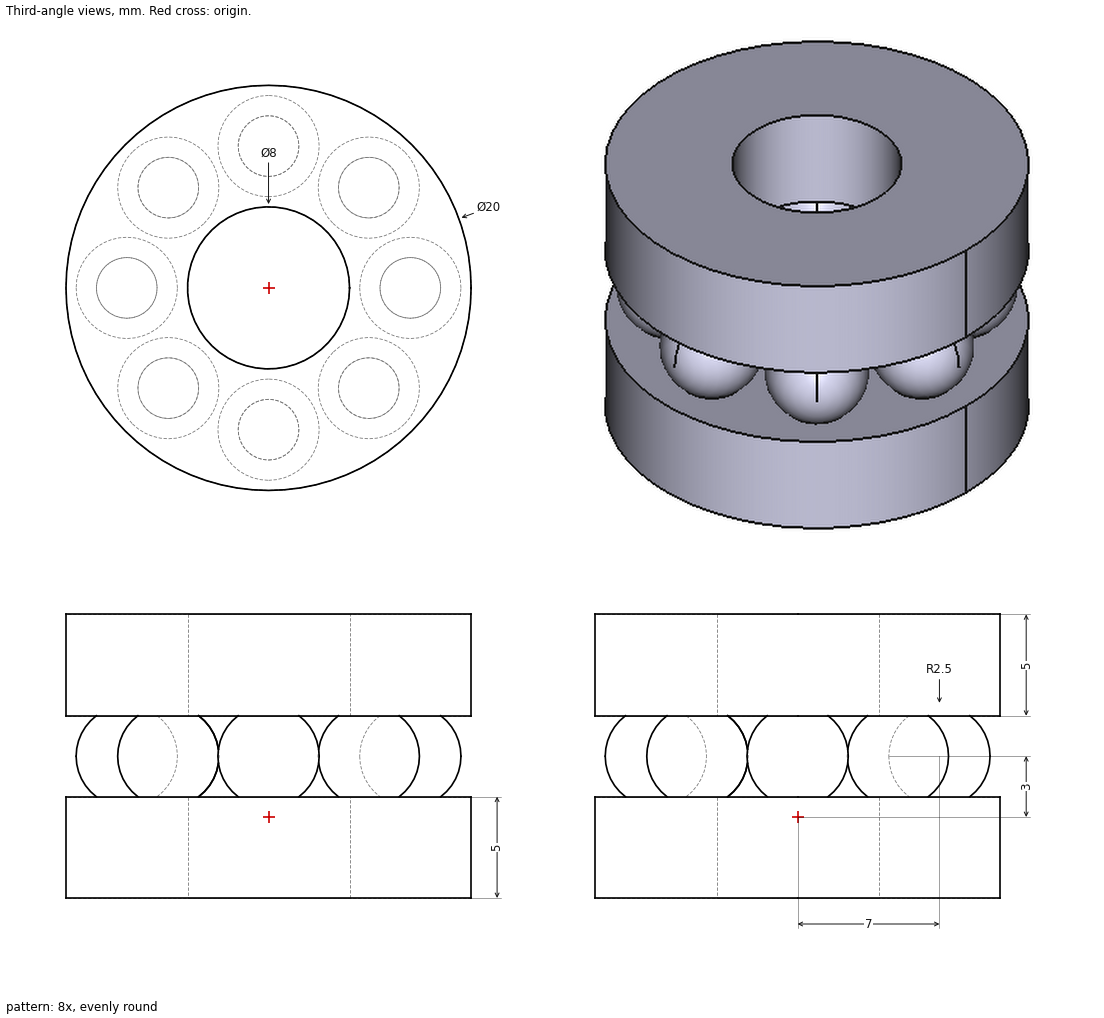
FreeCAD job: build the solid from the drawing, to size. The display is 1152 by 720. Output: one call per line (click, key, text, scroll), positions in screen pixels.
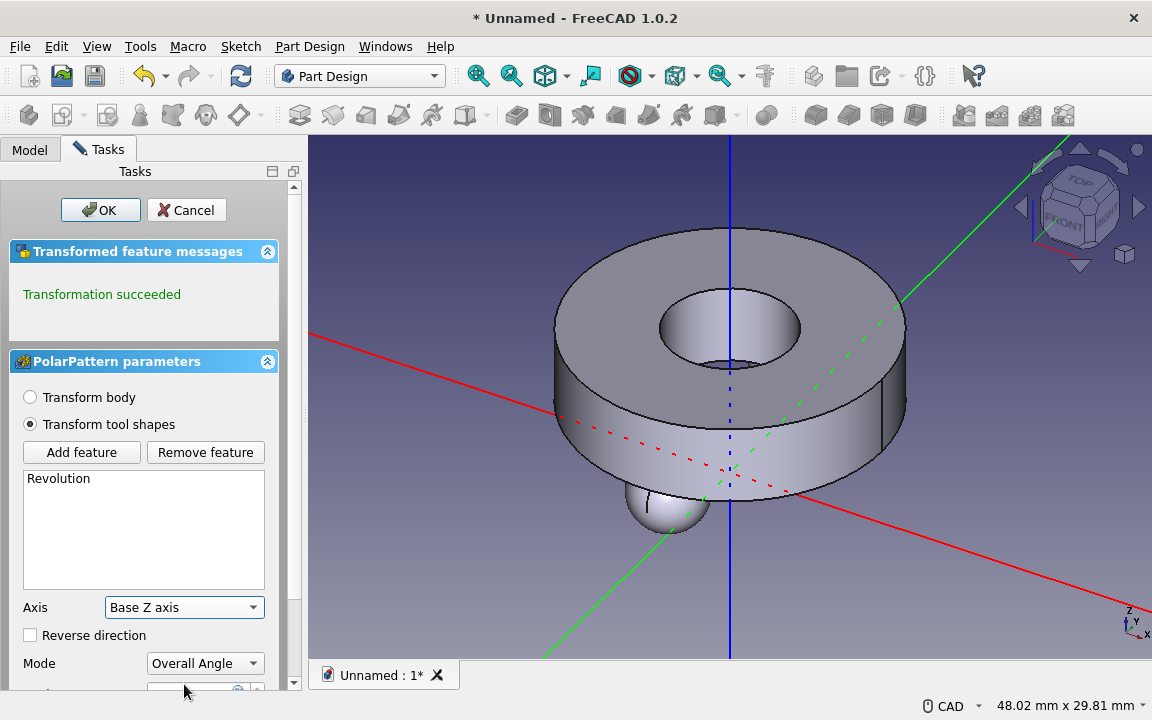
scroll(294, 436, down, 2)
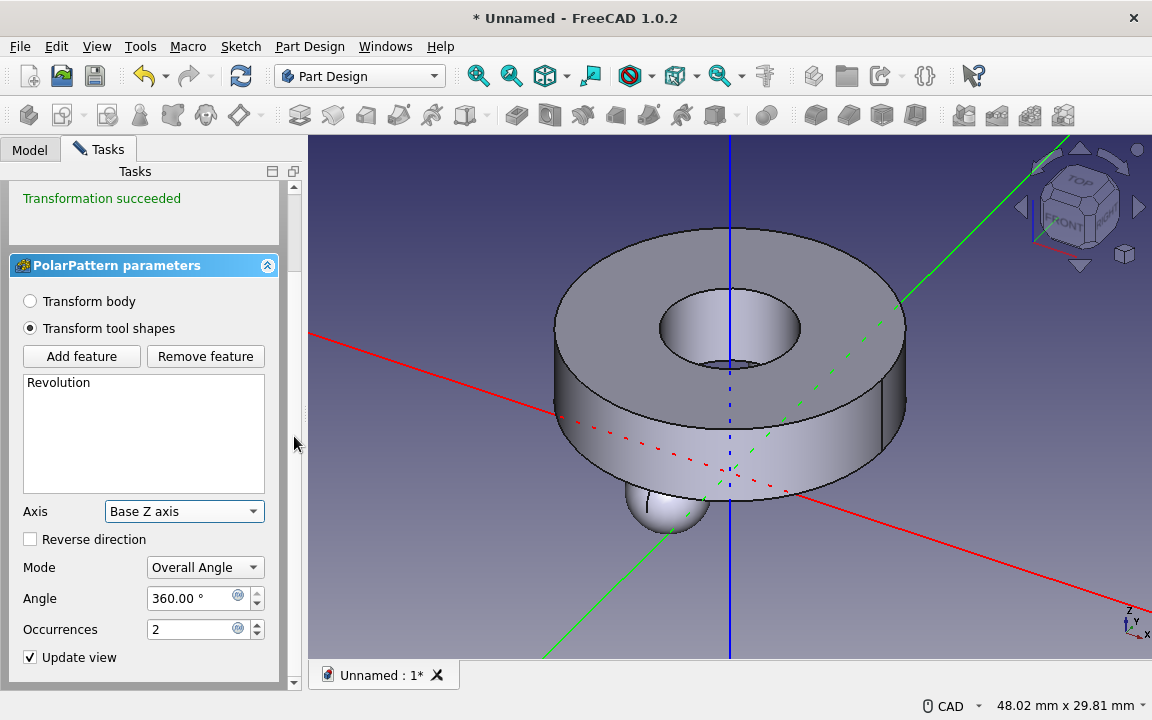
triple_click(199, 630)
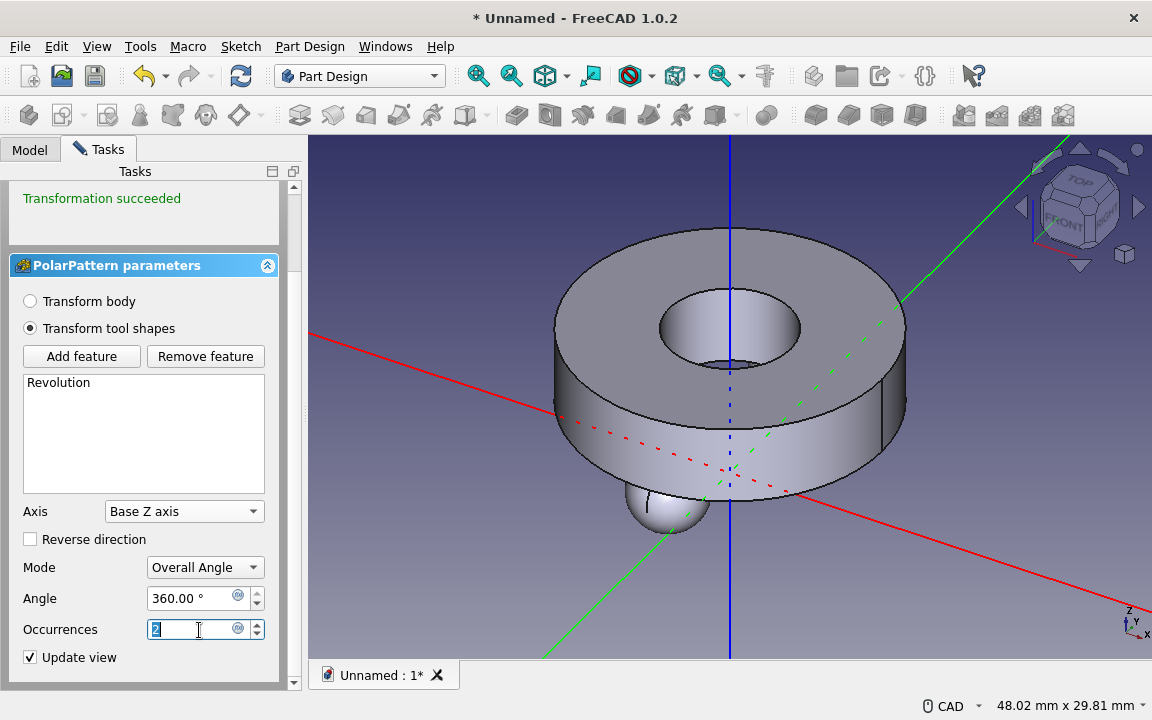
text(8)
key(Tab)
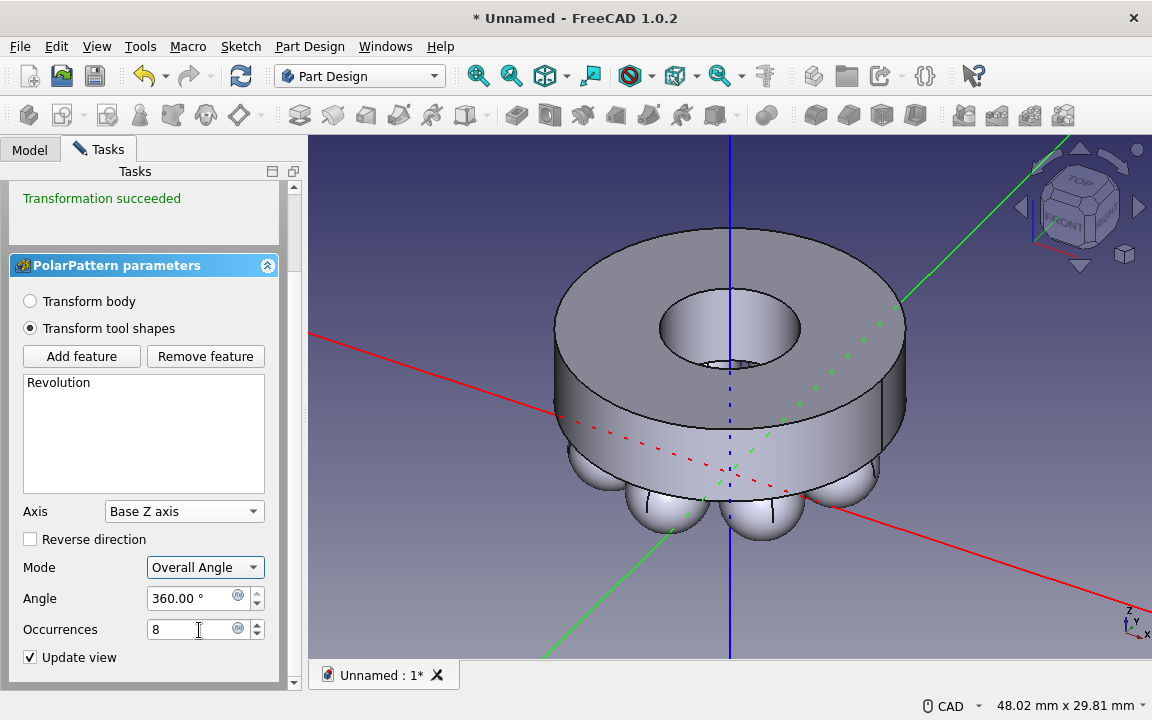
scroll(294, 436, up, 3)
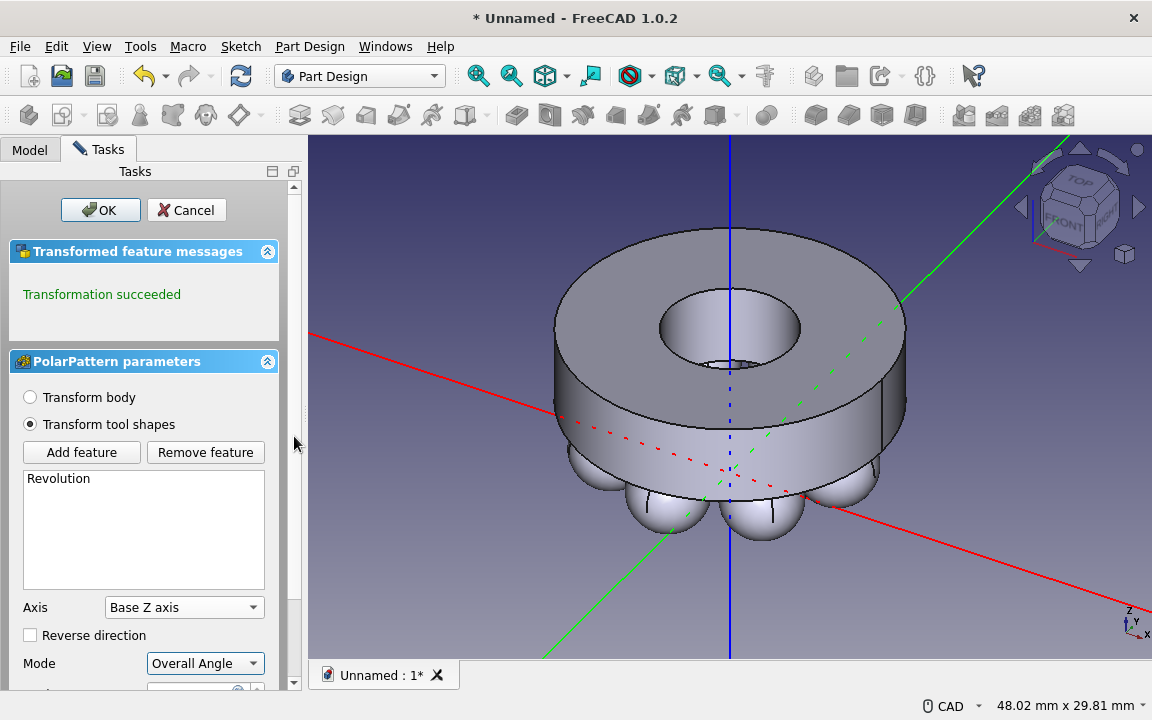
click(101, 210)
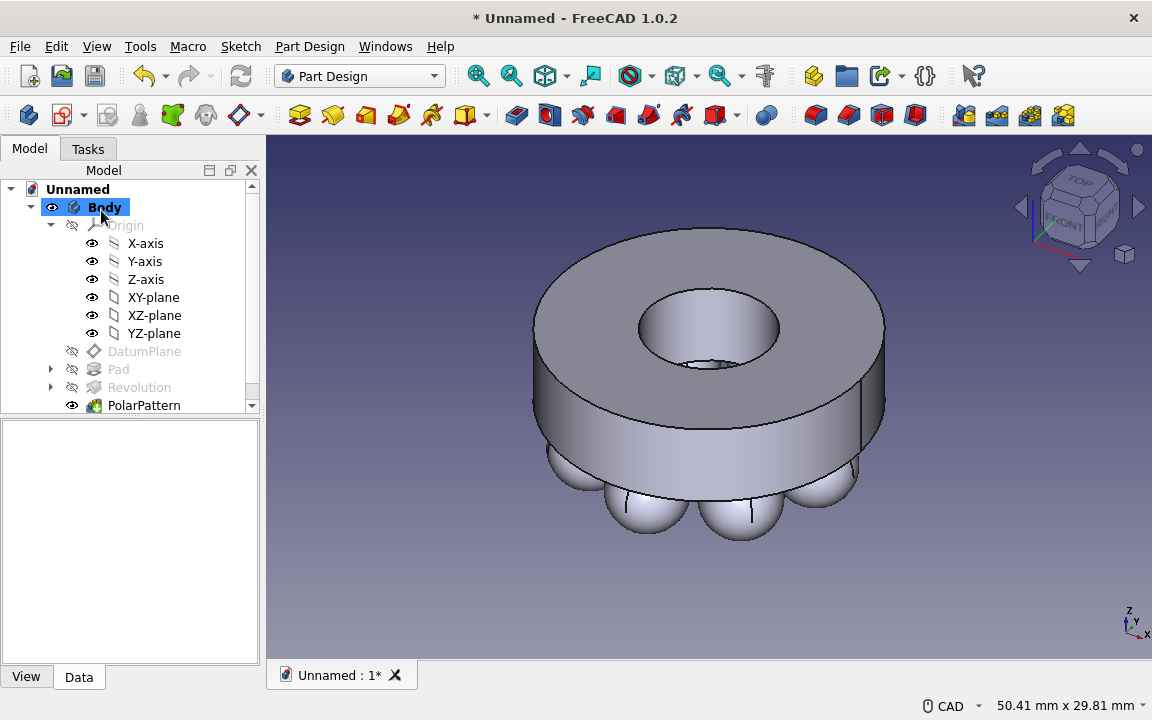
click(137, 297)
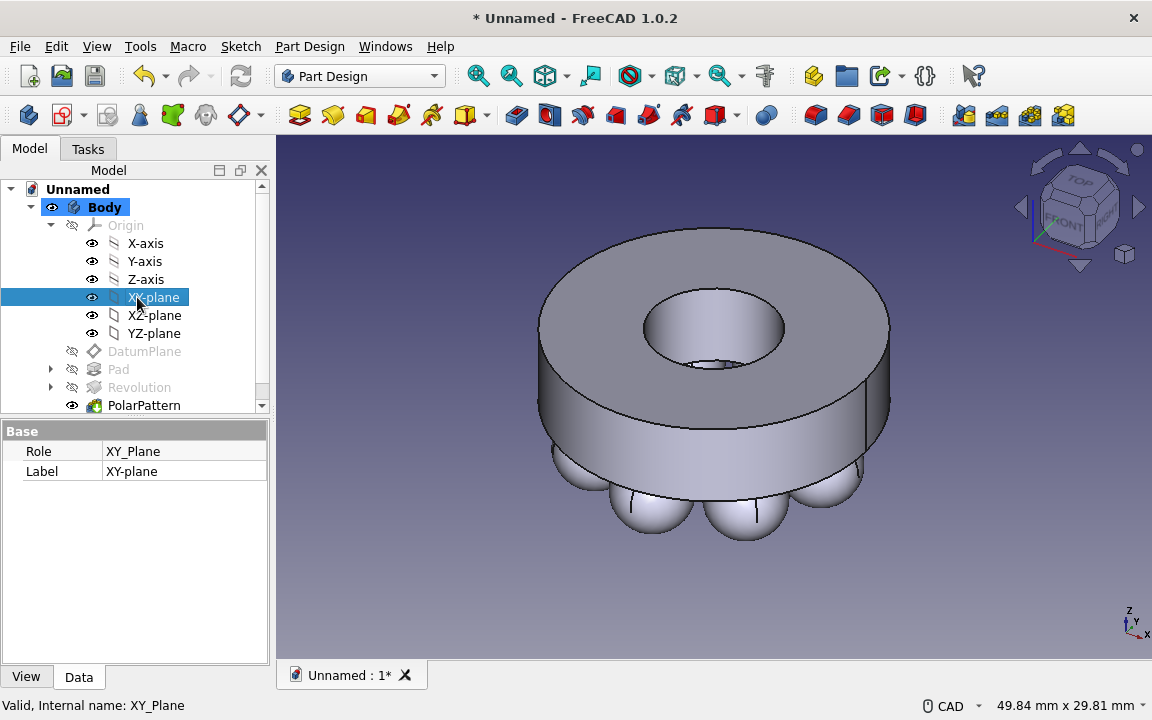
click(238, 116)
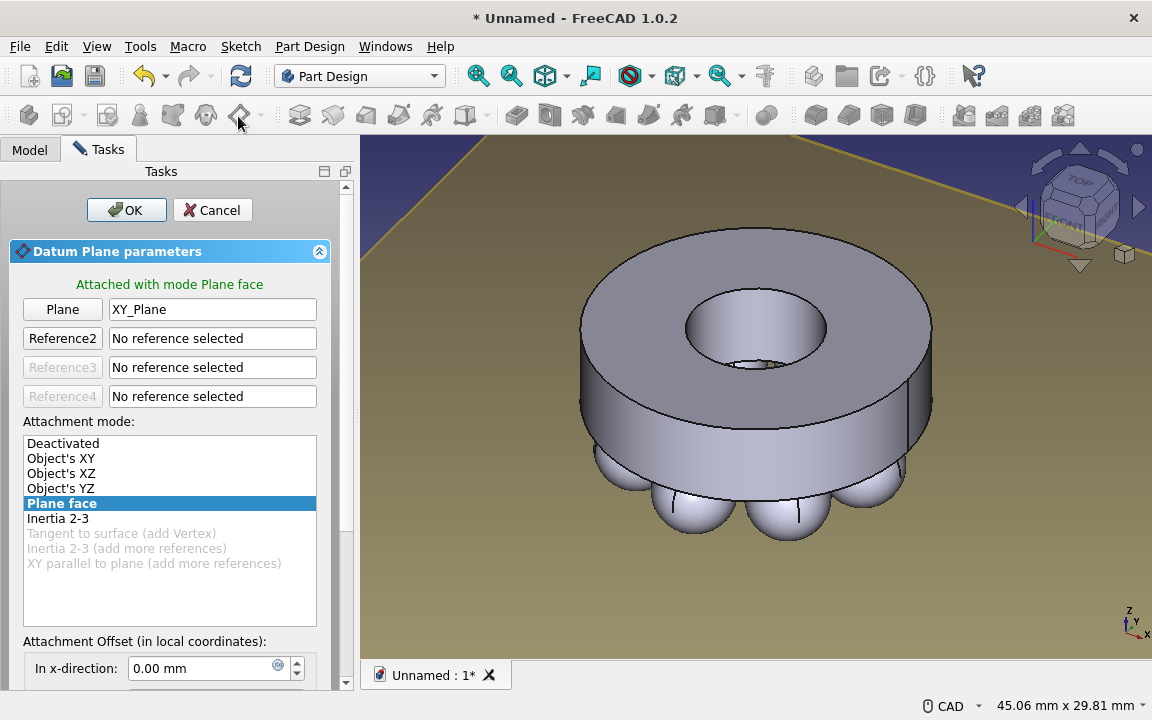
scroll(346, 436, down, 2)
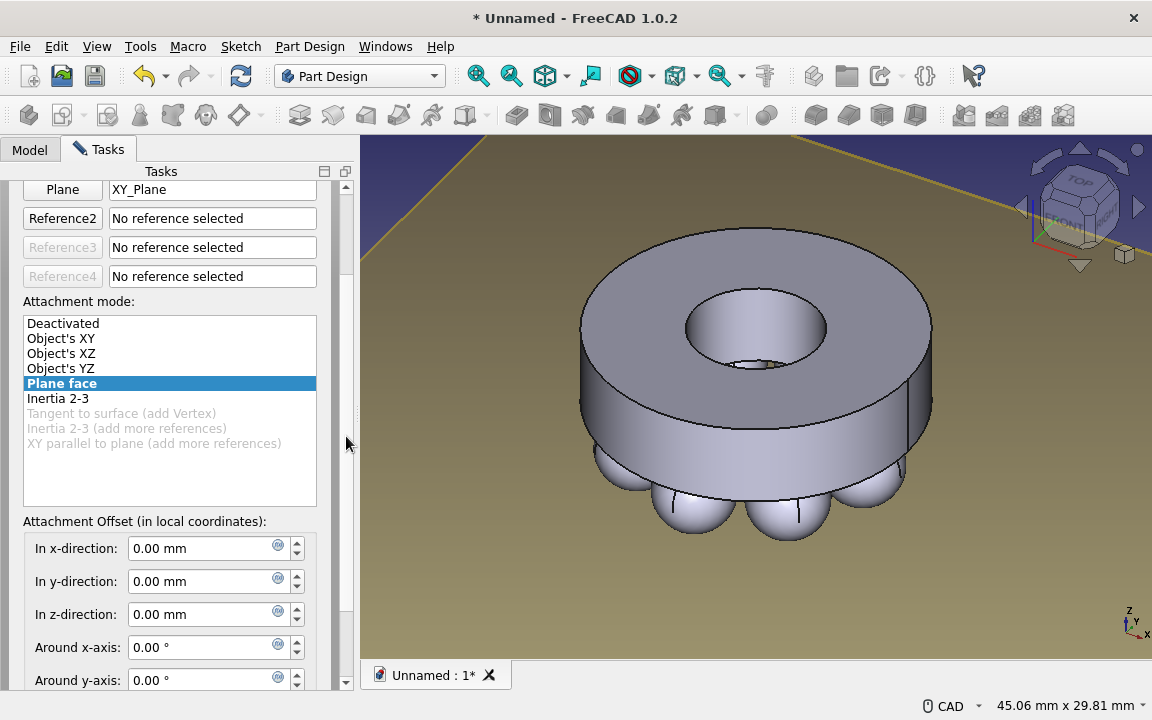
triple_click(210, 614)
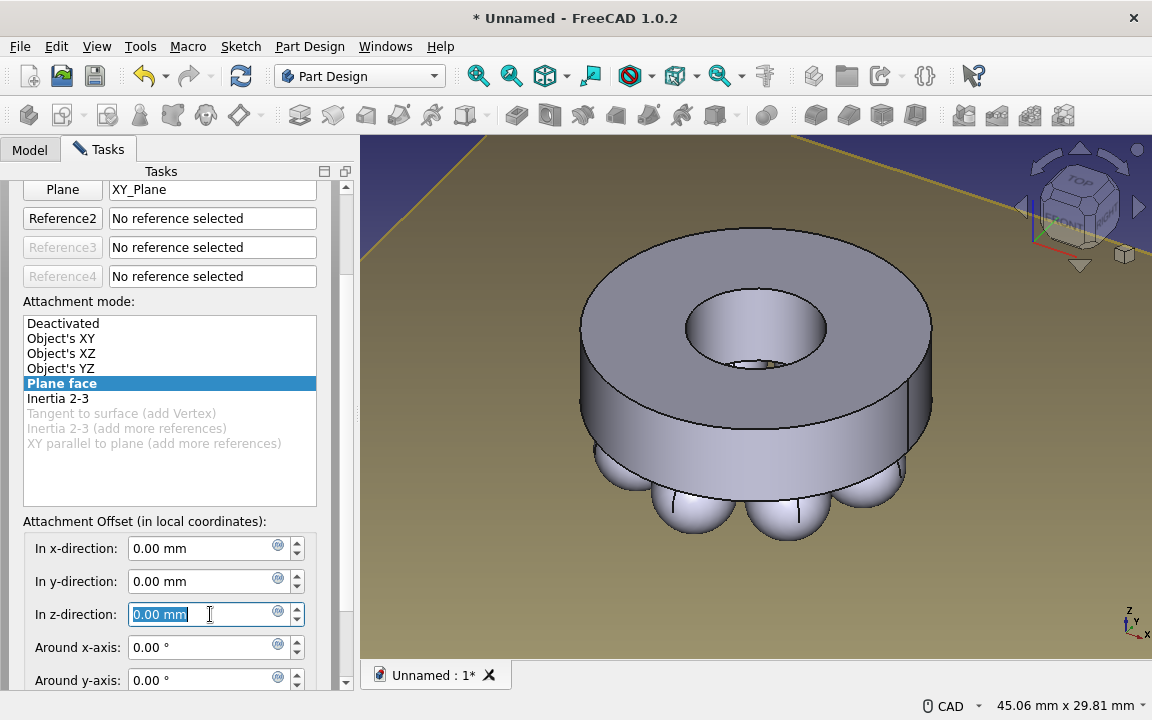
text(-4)
key(Tab)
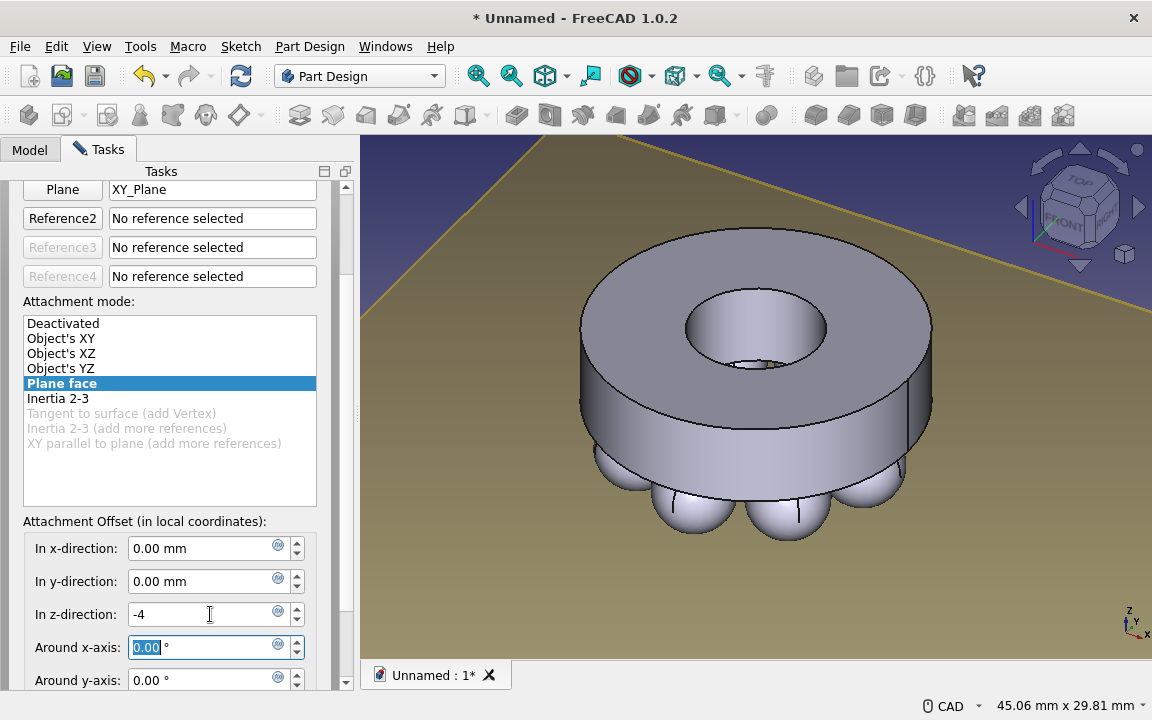
scroll(346, 436, up, 3)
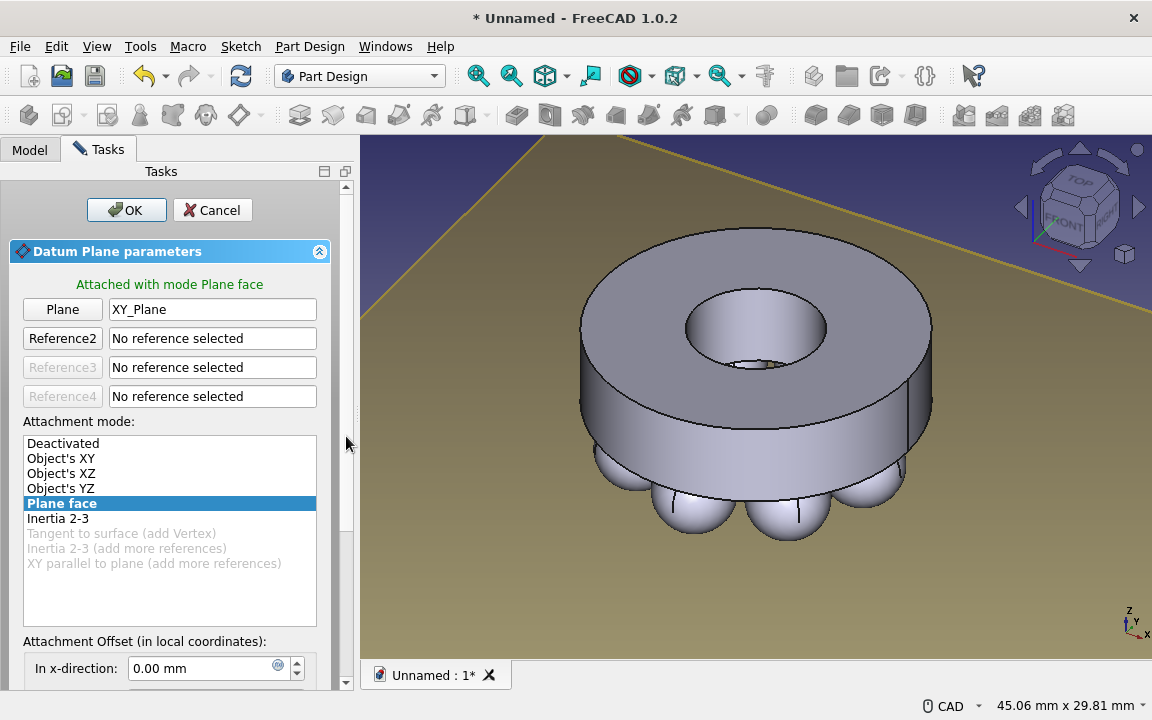
click(127, 210)